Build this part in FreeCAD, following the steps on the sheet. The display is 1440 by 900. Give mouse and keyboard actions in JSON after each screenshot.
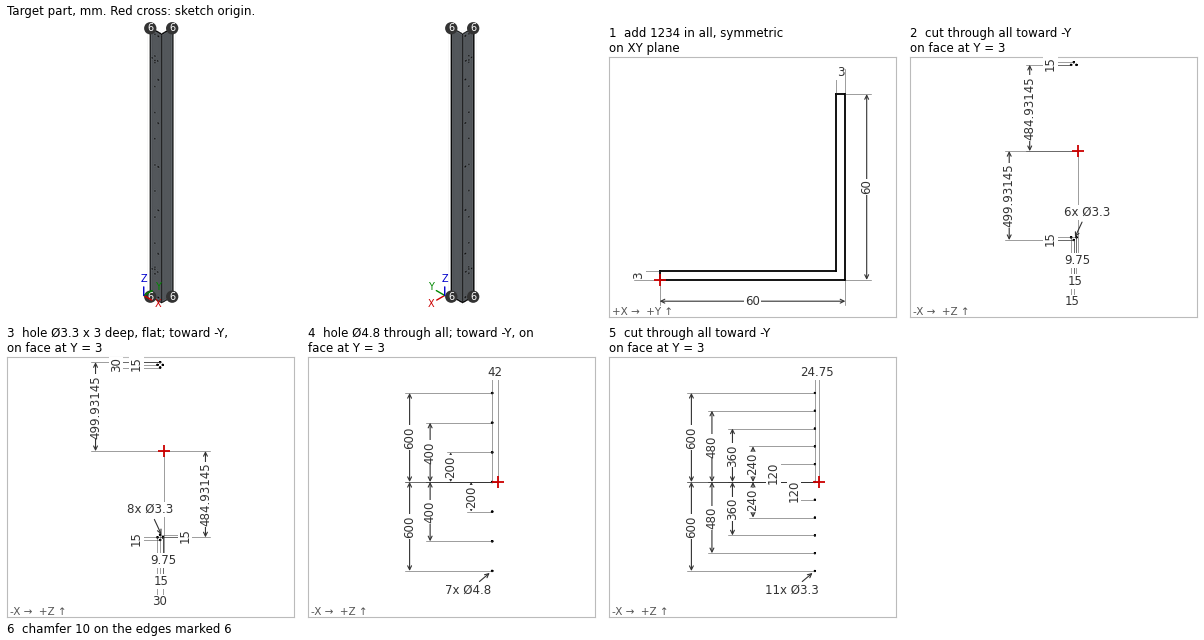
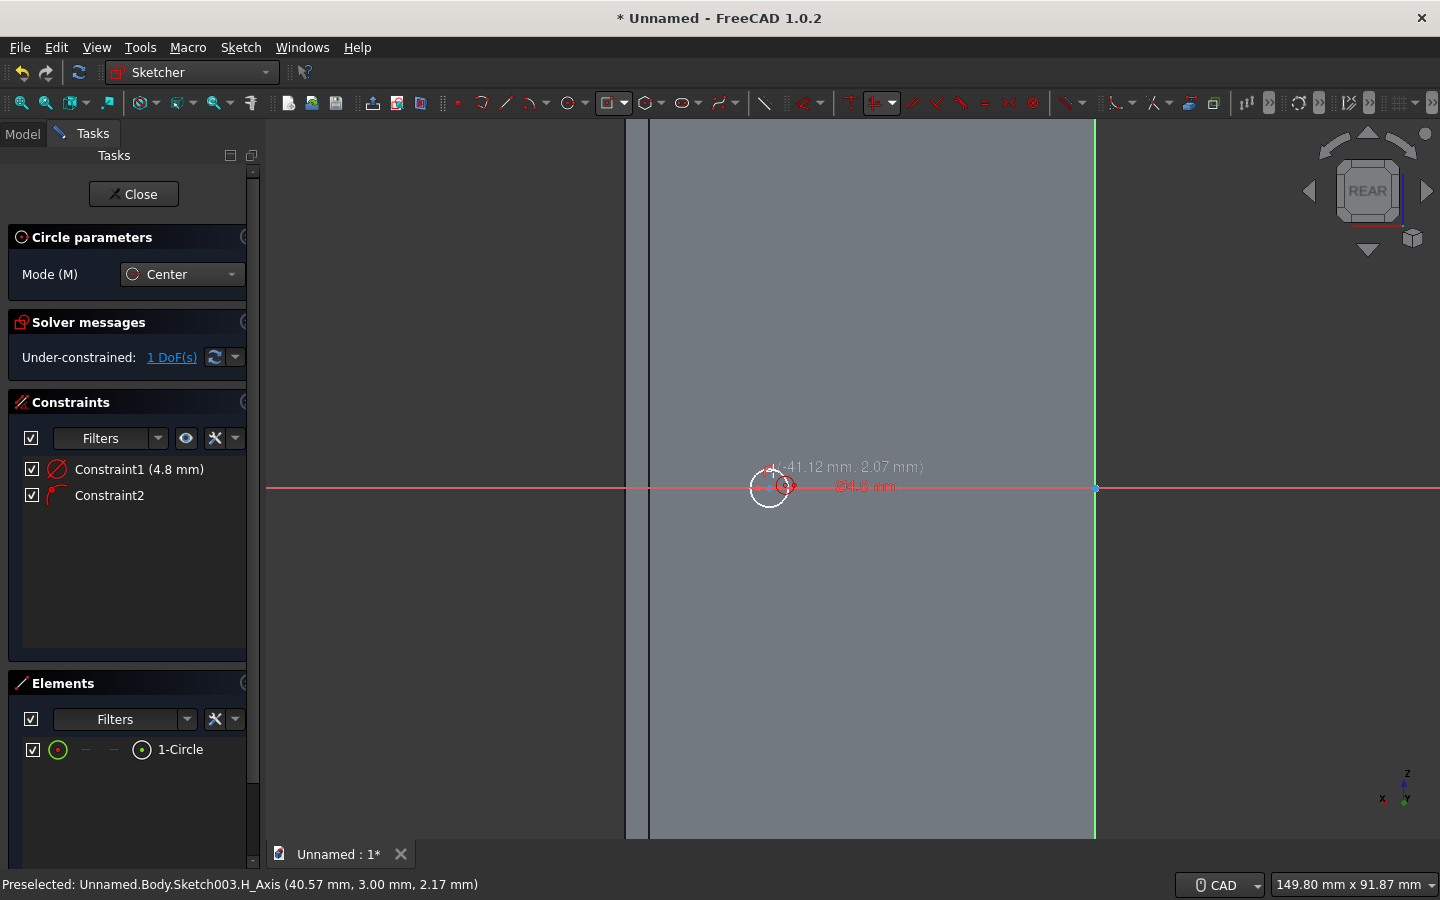
{"action": "scroll", "coordinate": [777, 479], "scroll_direction": "down", "scroll_amount": 15}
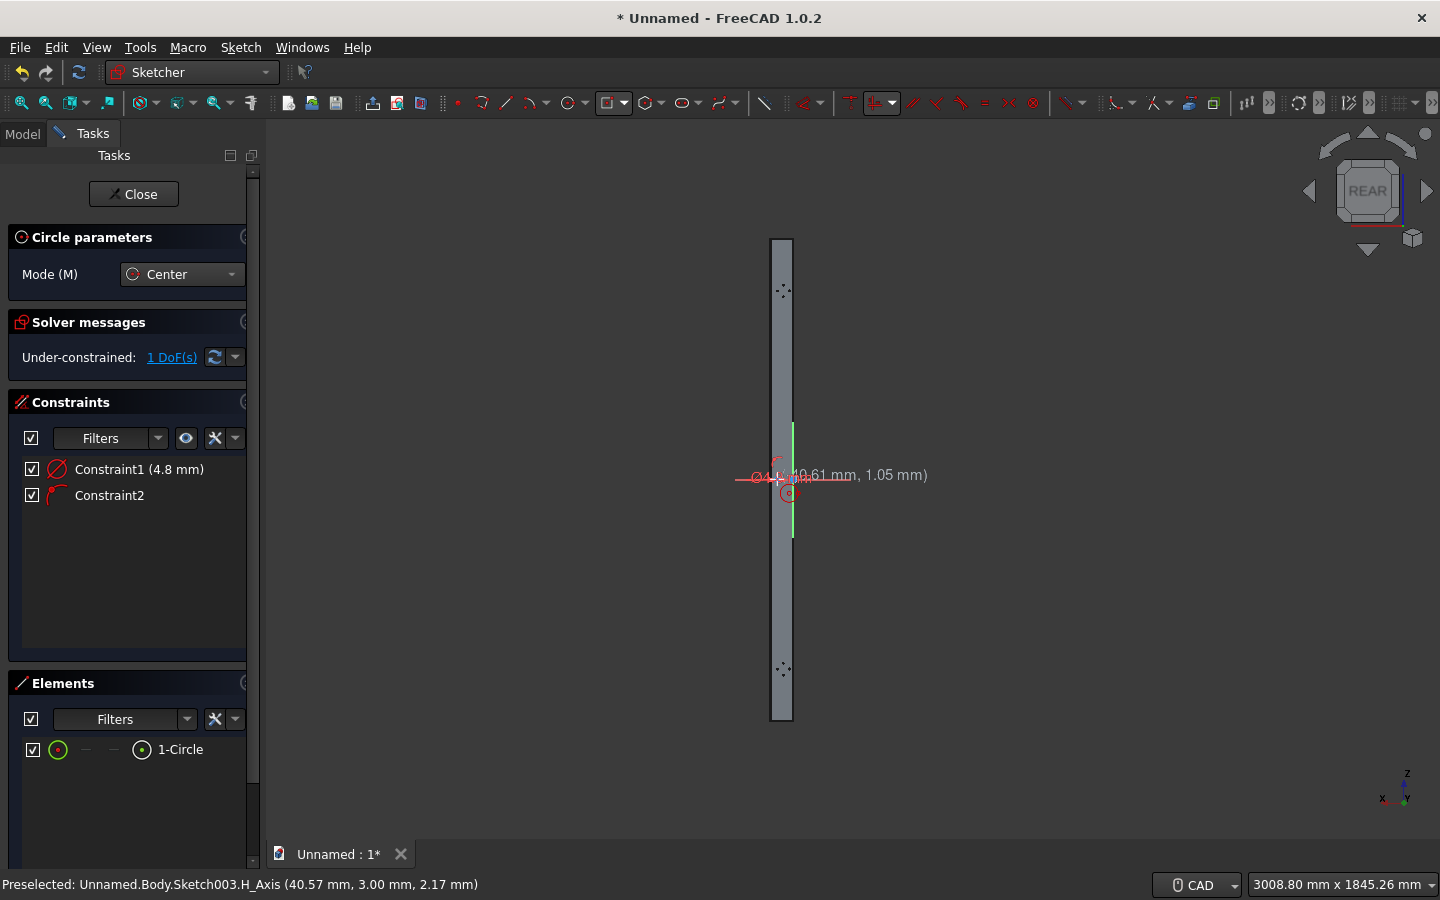
{"action": "scroll", "coordinate": [777, 558], "scroll_direction": "up", "scroll_amount": 16}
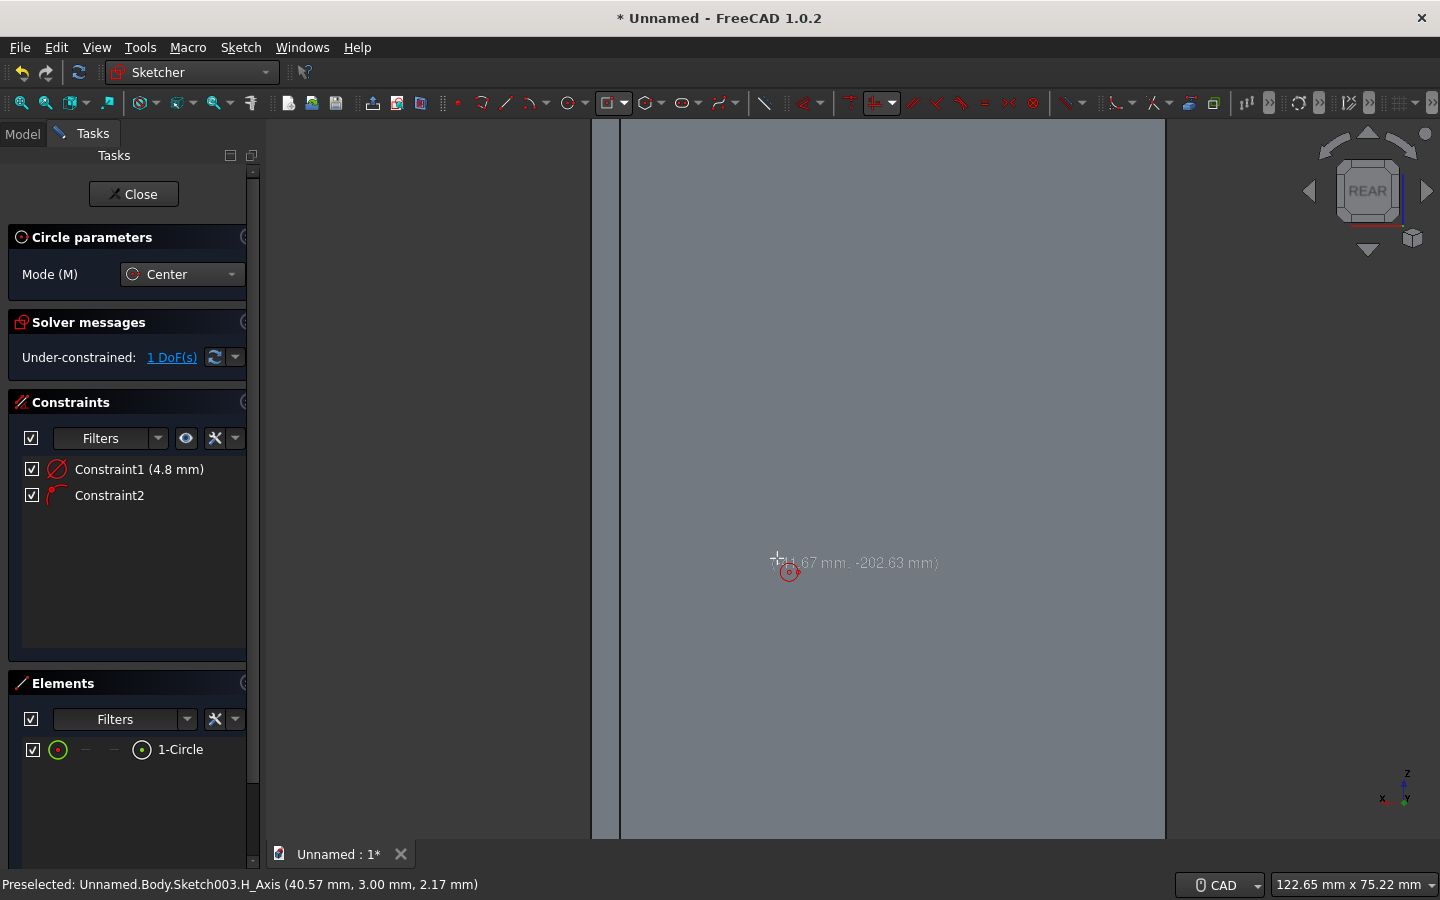
{"action": "scroll", "coordinate": [776, 576], "scroll_direction": "down", "scroll_amount": 15}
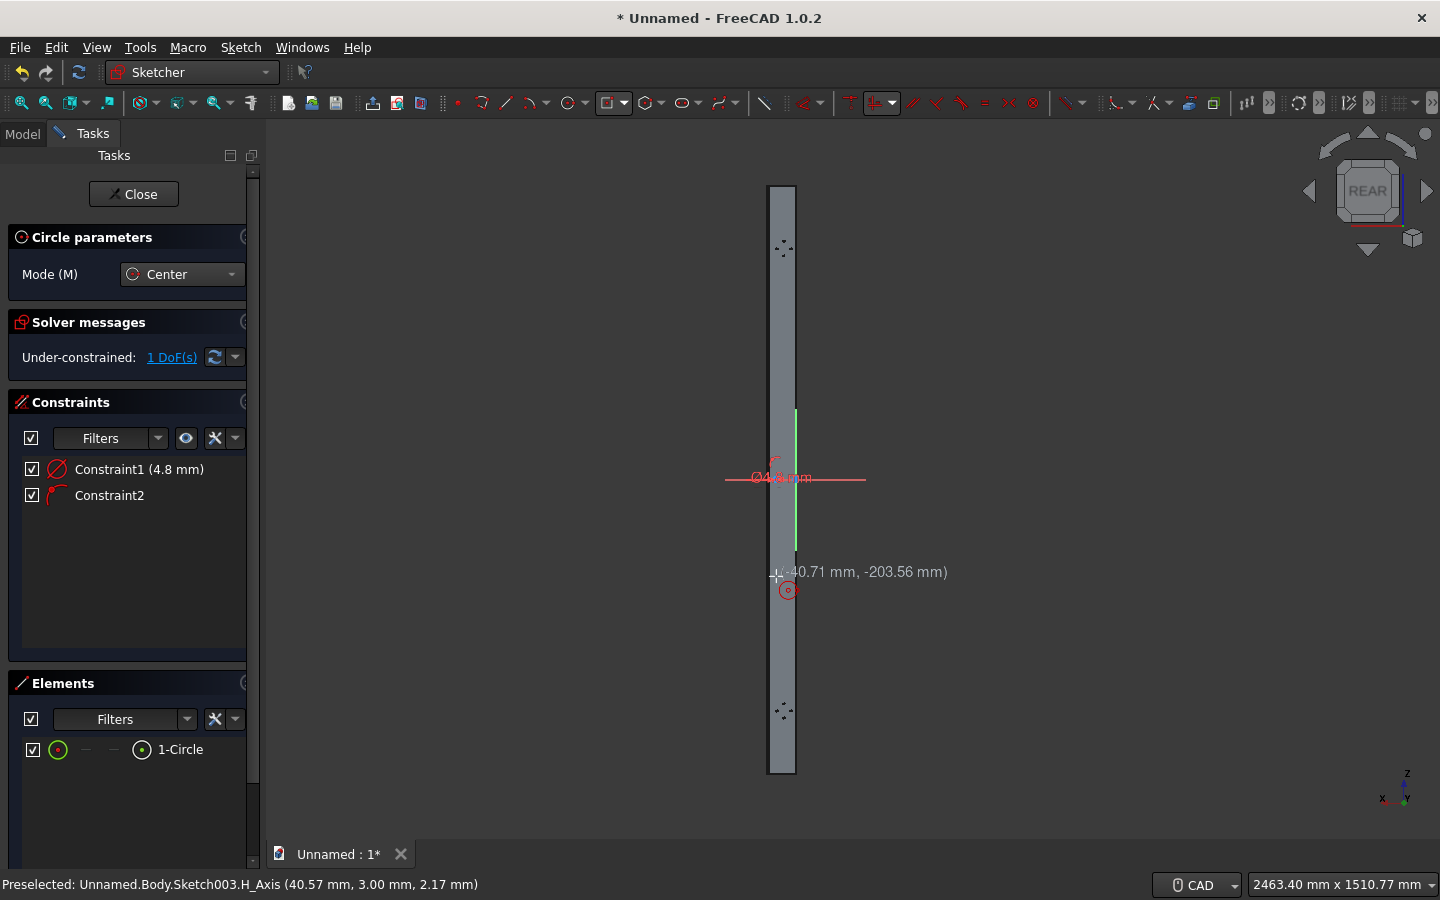
{"action": "left_click", "coordinate": [776, 575]}
{"action": "mouse_move", "coordinate": [777, 574]}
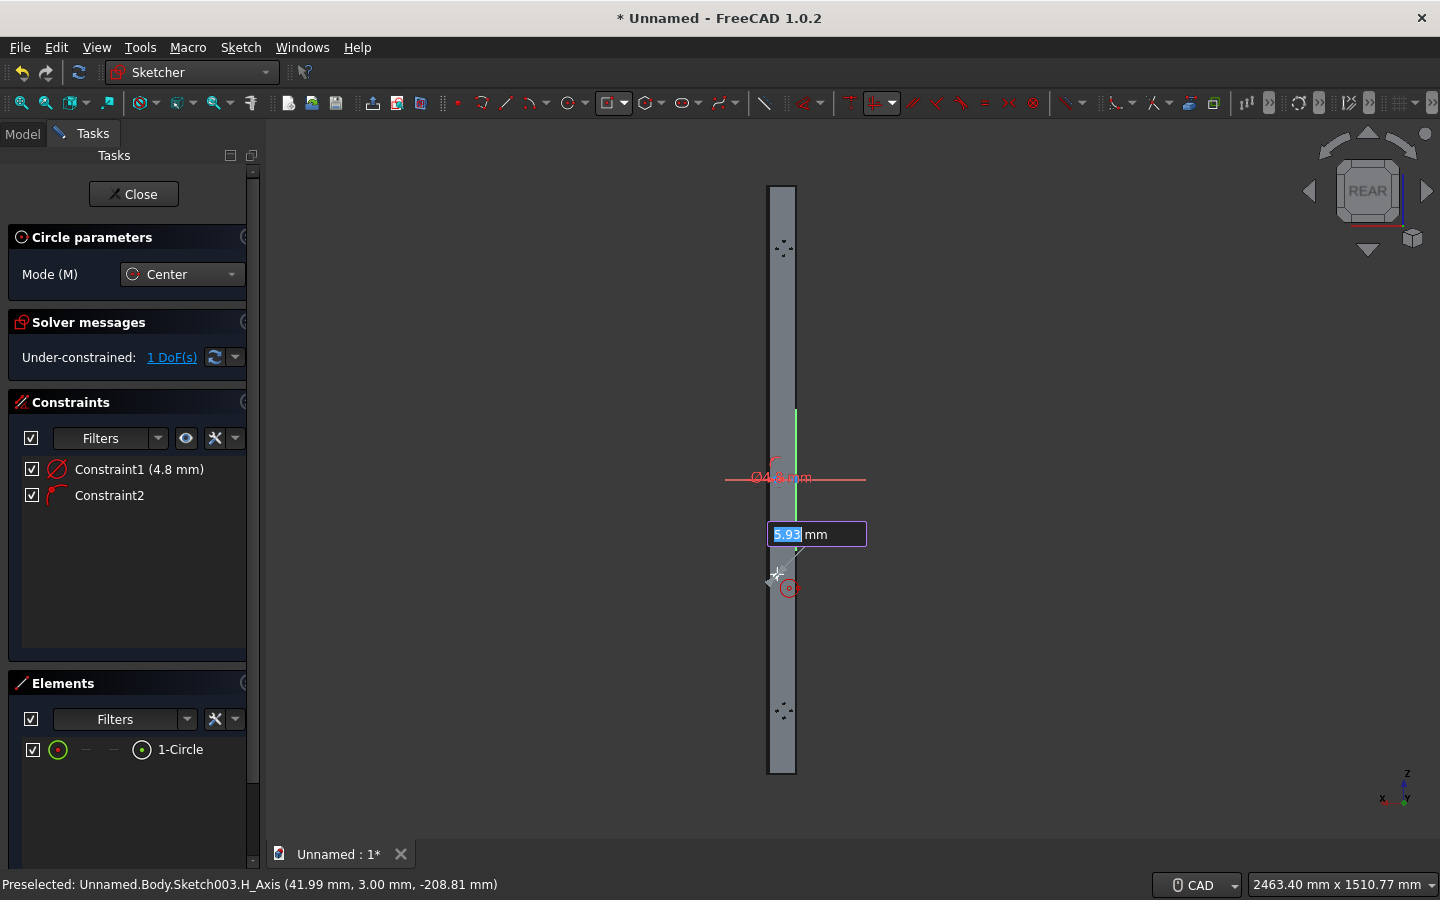
{"action": "type", "text": "4.8"}
{"action": "key", "text": "Return"}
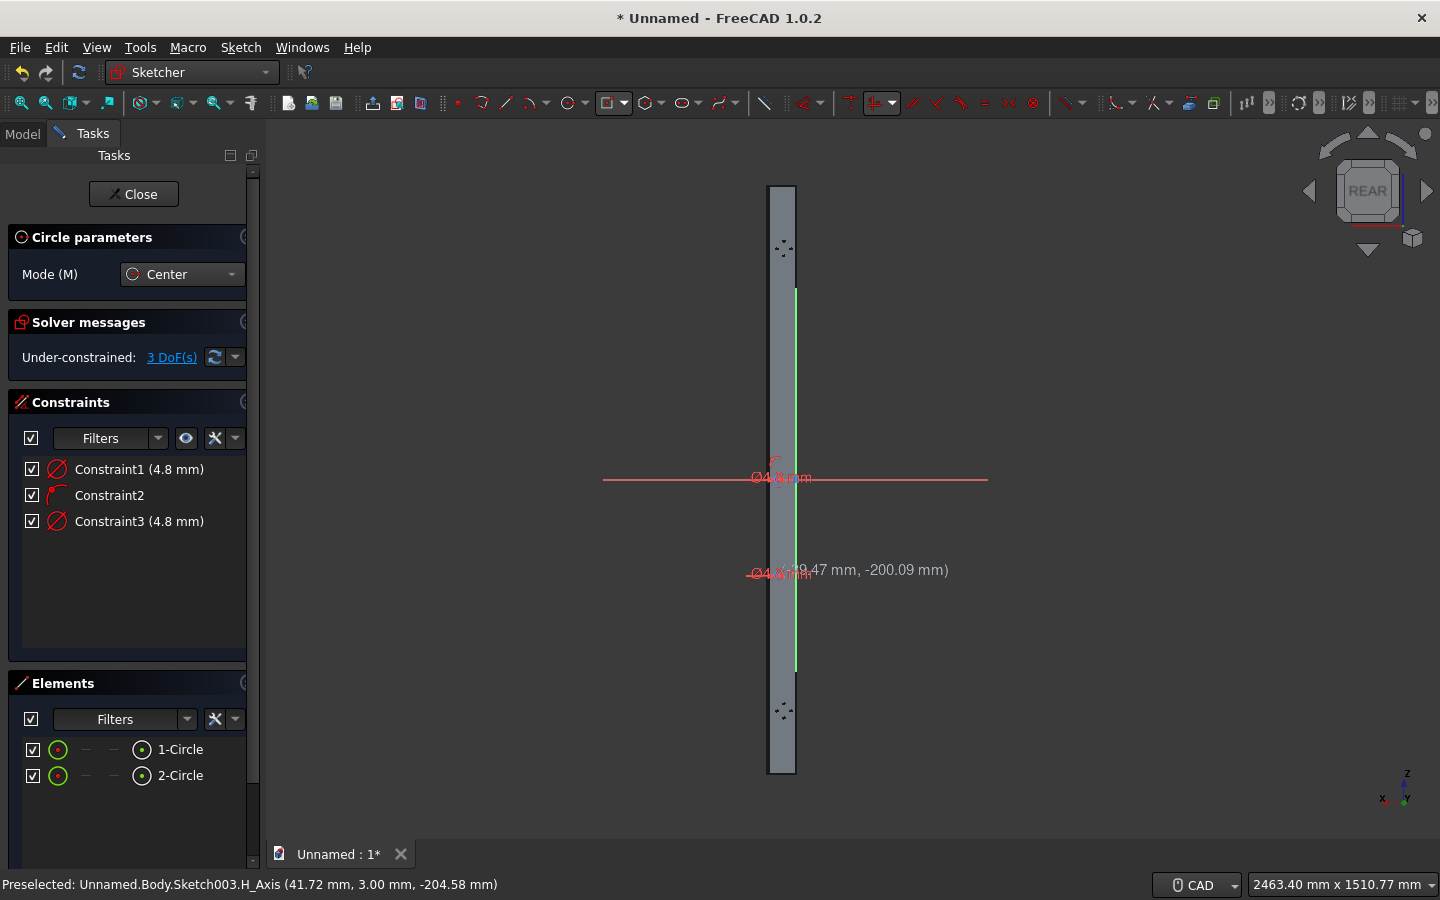
{"action": "scroll", "coordinate": [776, 670], "scroll_direction": "up", "scroll_amount": 15}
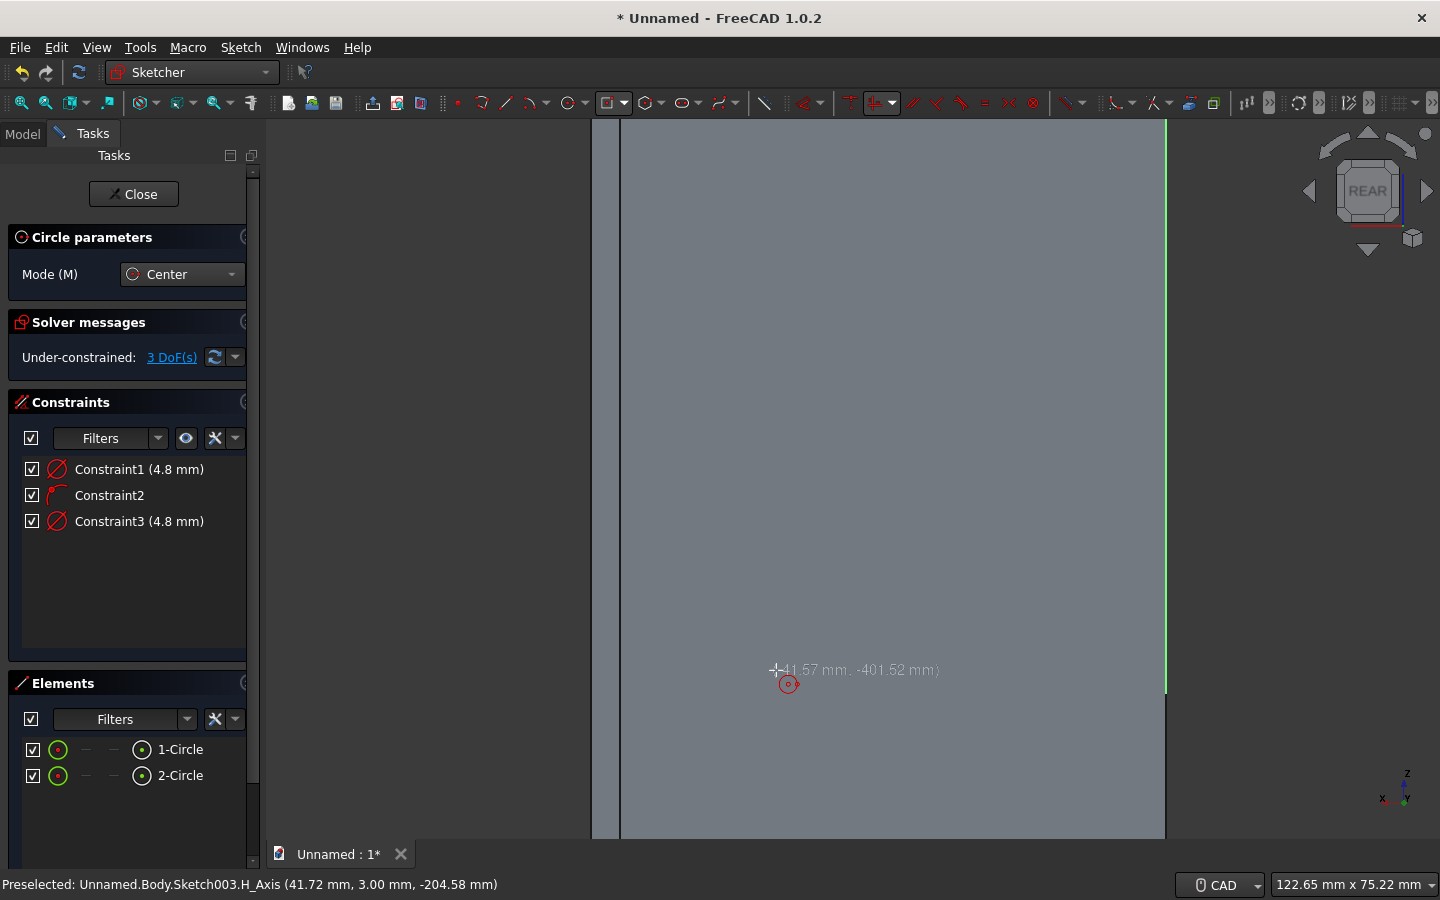
{"action": "scroll", "coordinate": [776, 670], "scroll_direction": "down", "scroll_amount": 15}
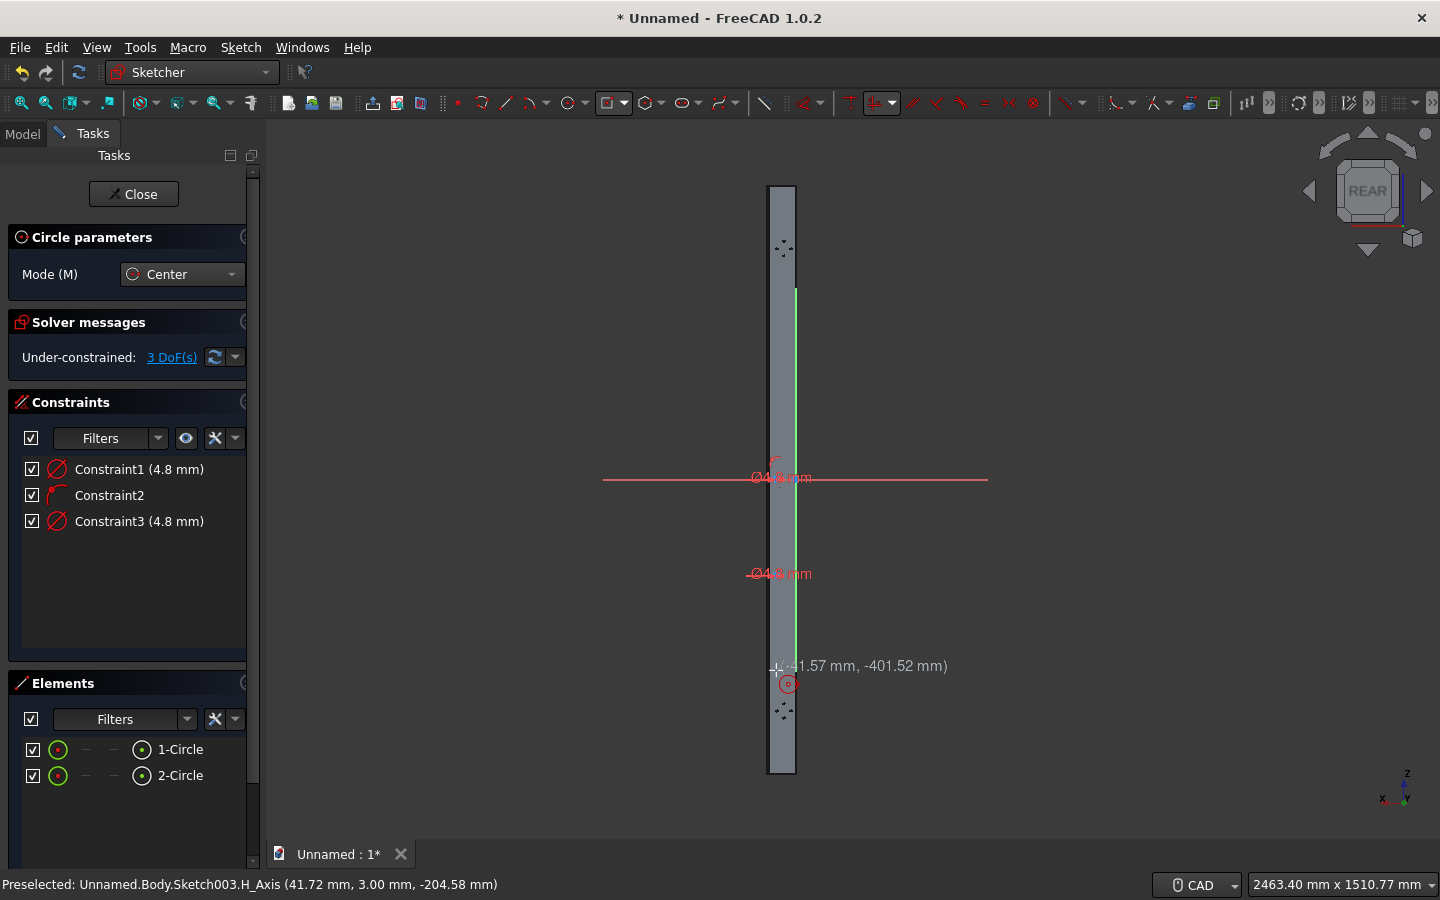
{"action": "left_click", "coordinate": [776, 670]}
{"action": "mouse_move", "coordinate": [777, 669]}